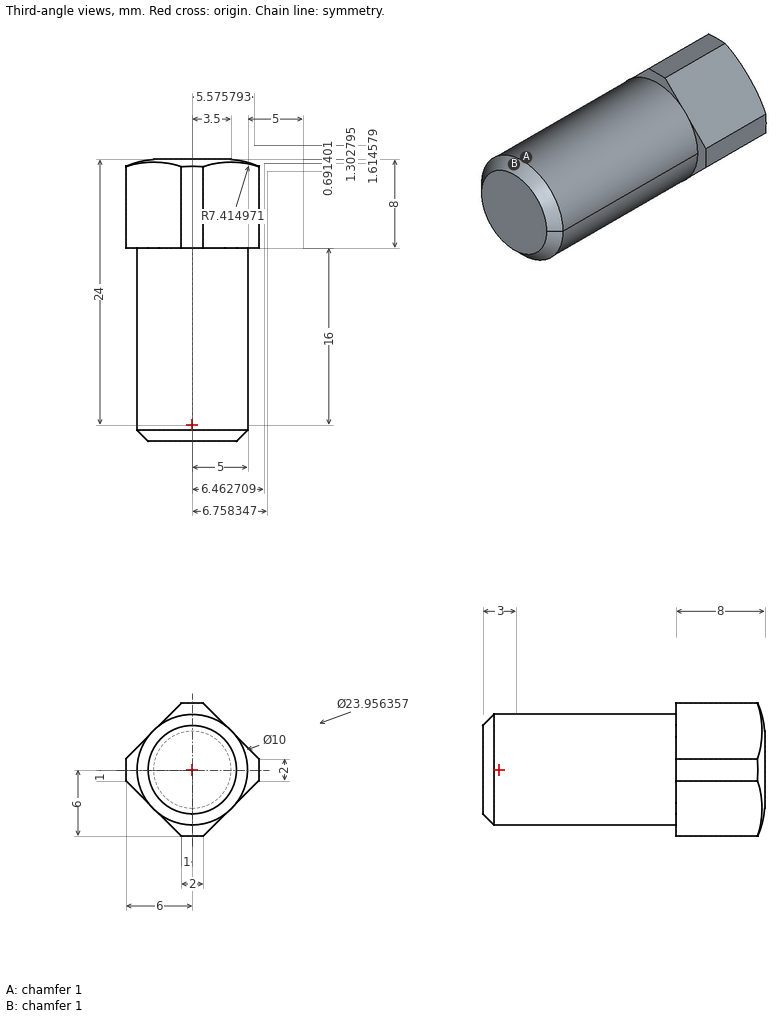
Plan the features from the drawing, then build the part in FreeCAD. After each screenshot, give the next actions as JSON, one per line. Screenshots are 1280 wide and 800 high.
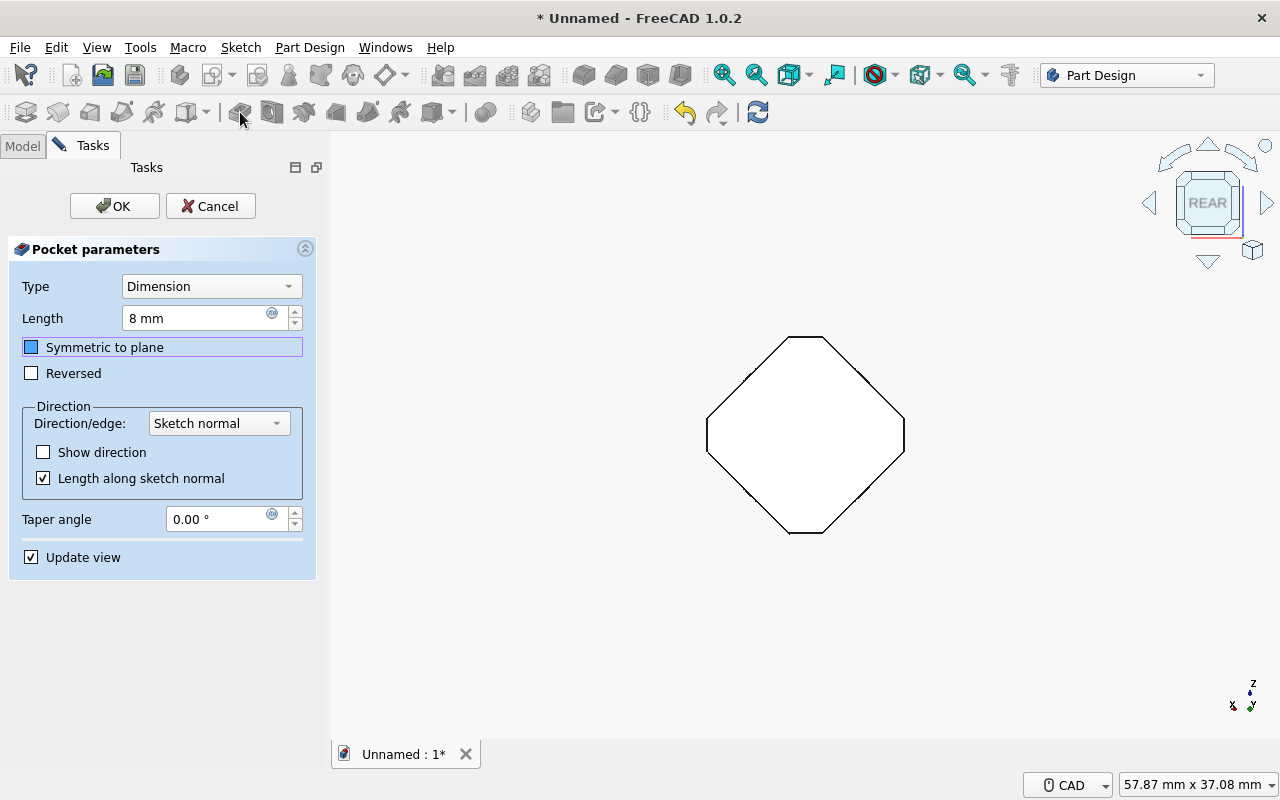
{"action": "left_click", "coordinate": [115, 206]}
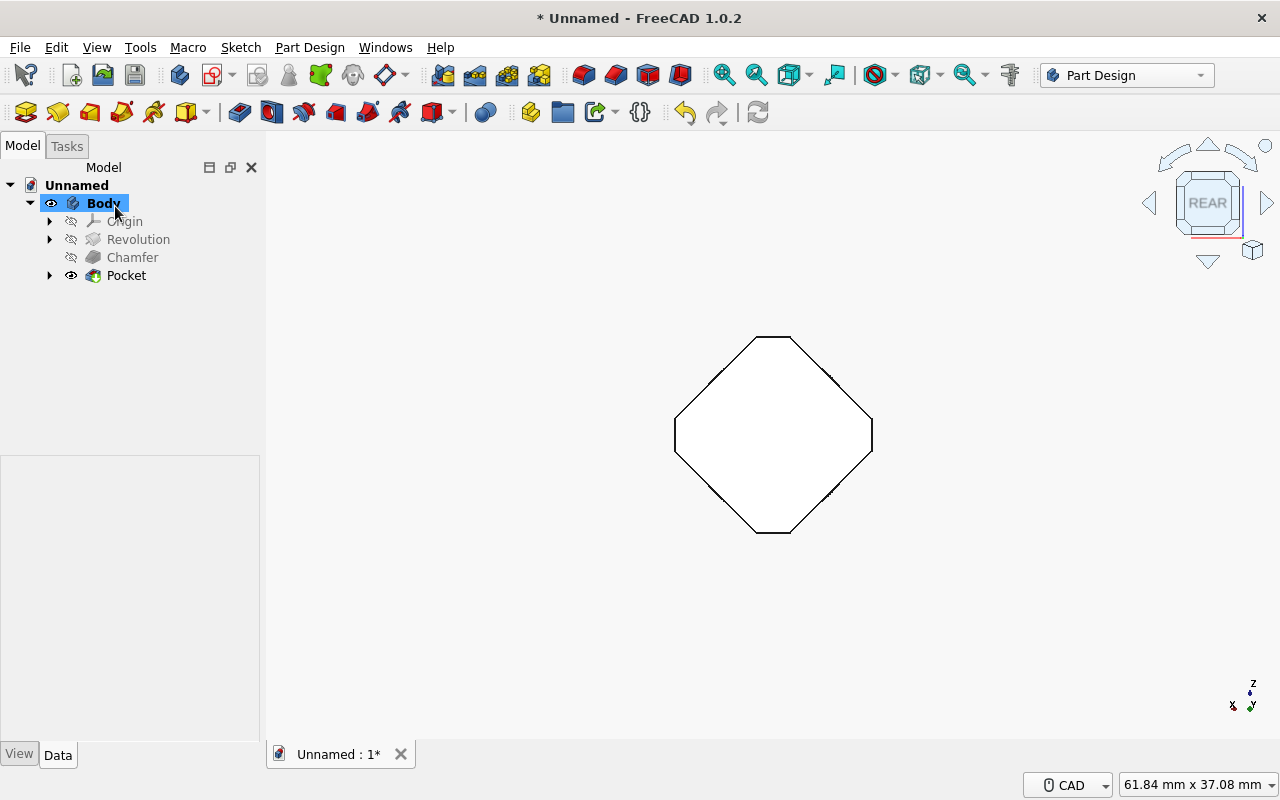
{"action": "left_click", "coordinate": [726, 76]}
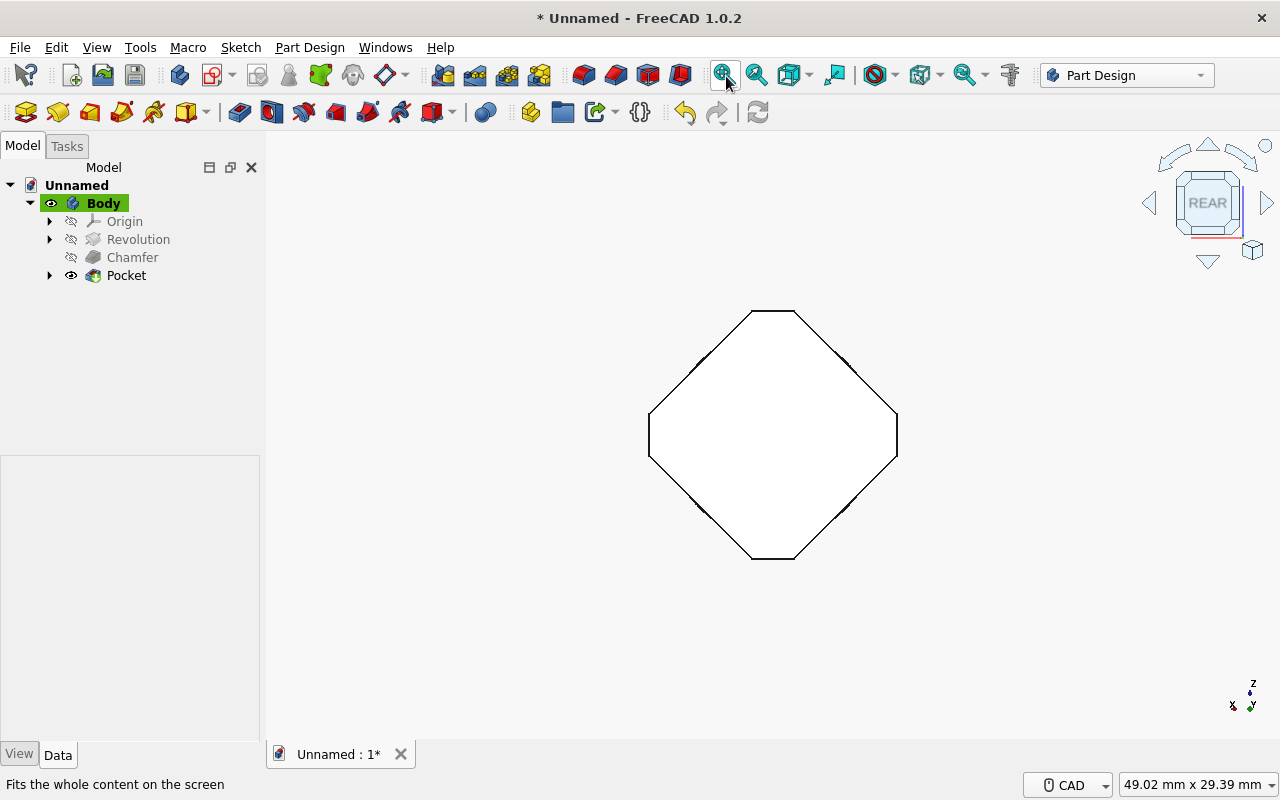
{"action": "left_click", "coordinate": [212, 76]}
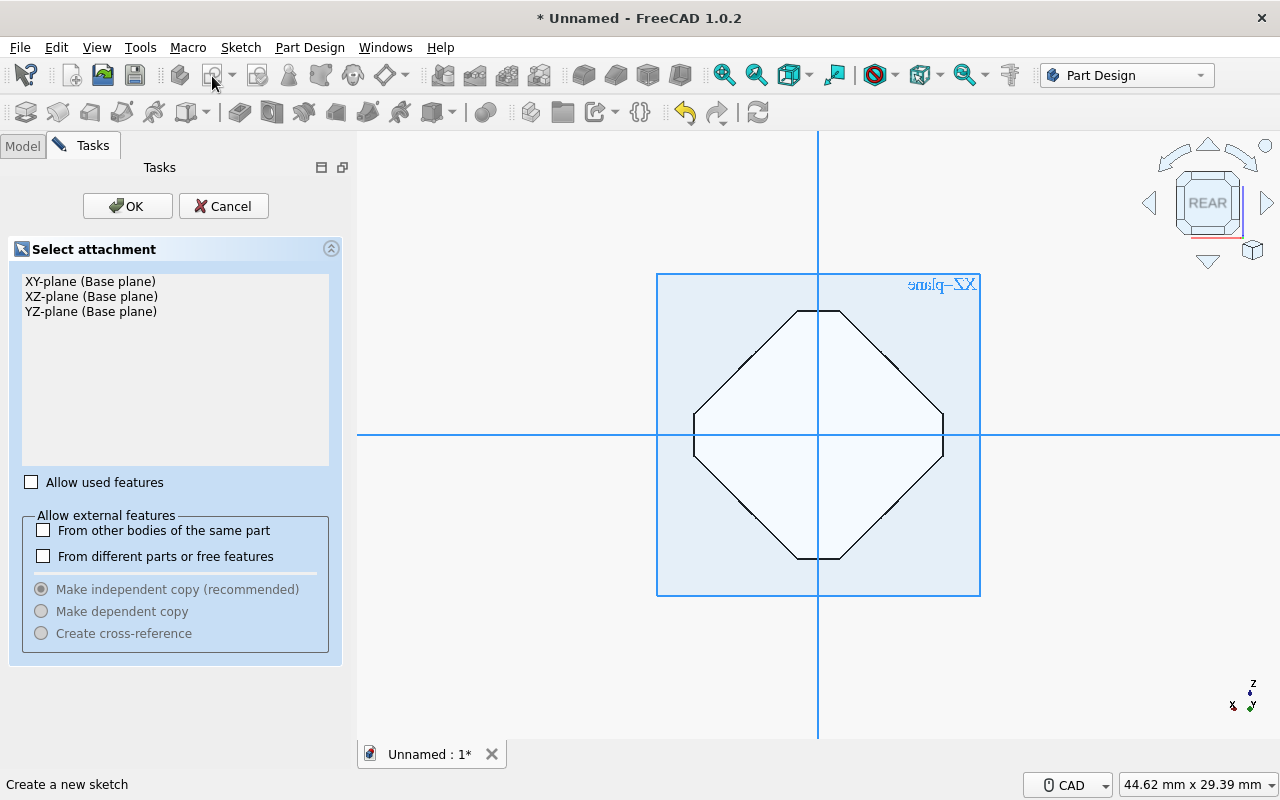
{"action": "left_click", "coordinate": [82, 282]}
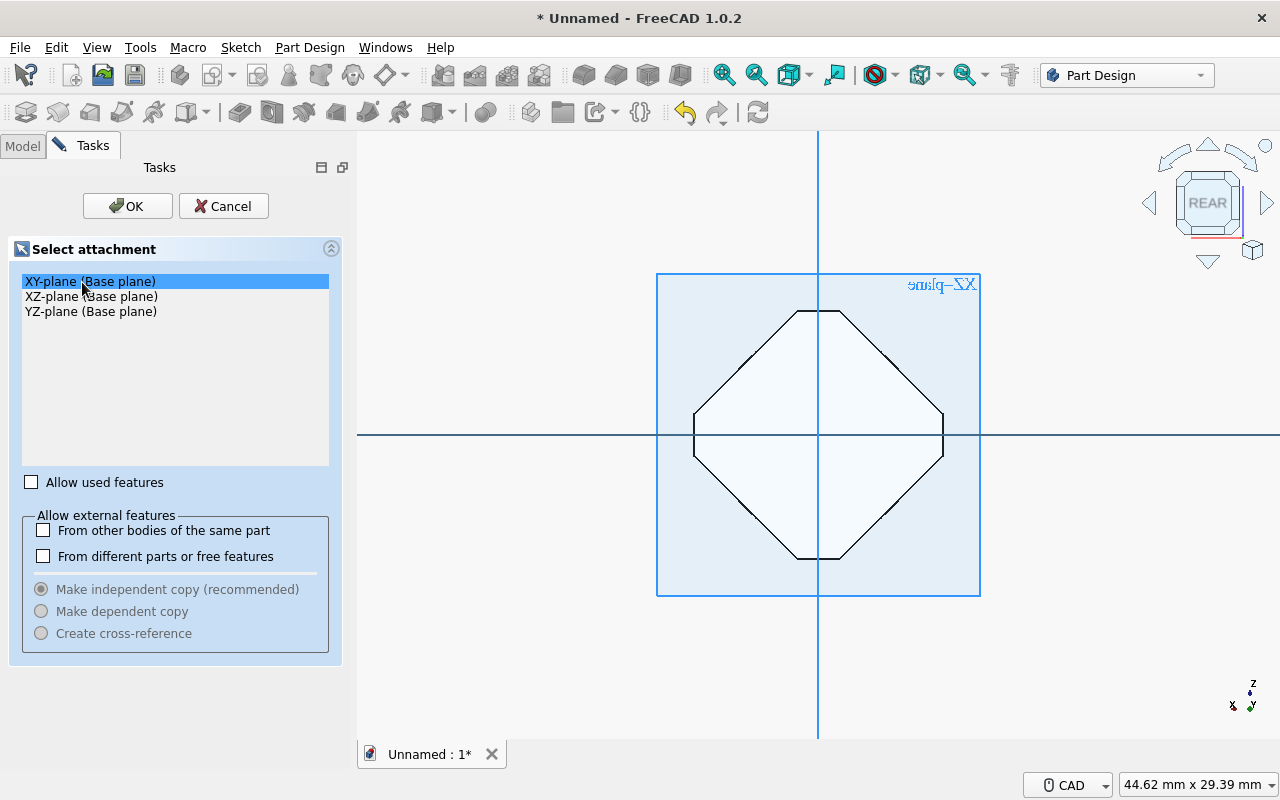
{"action": "left_click", "coordinate": [128, 206]}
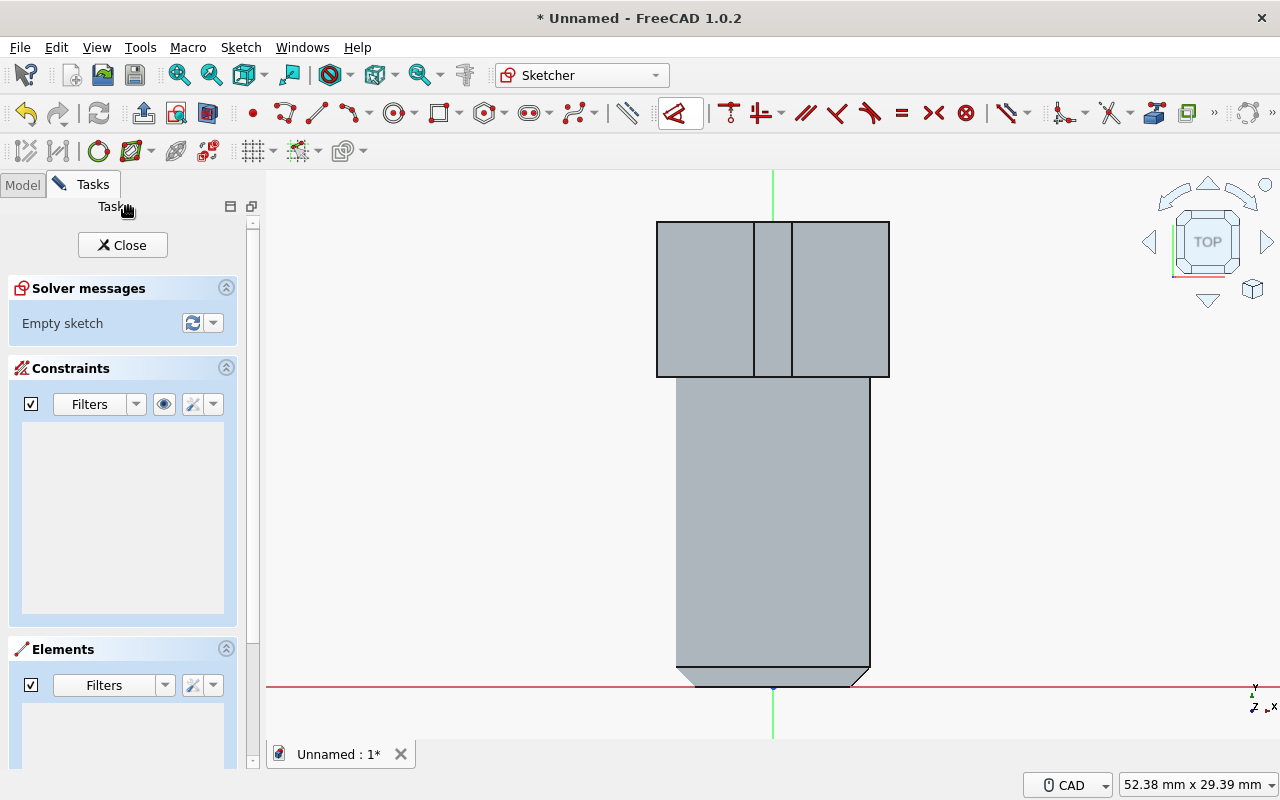
{"action": "left_click", "coordinate": [208, 114]}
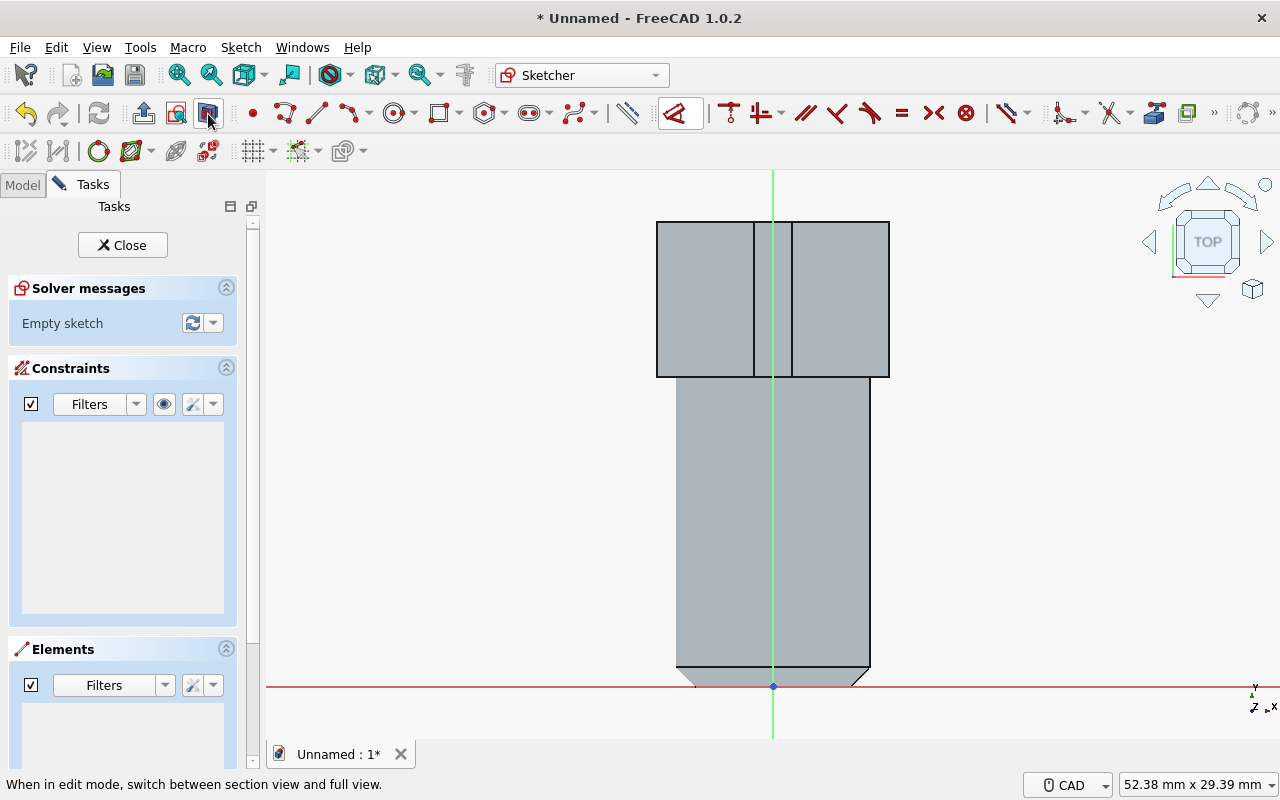
{"action": "scroll", "coordinate": [704, 454], "scroll_direction": "down", "scroll_amount": 5}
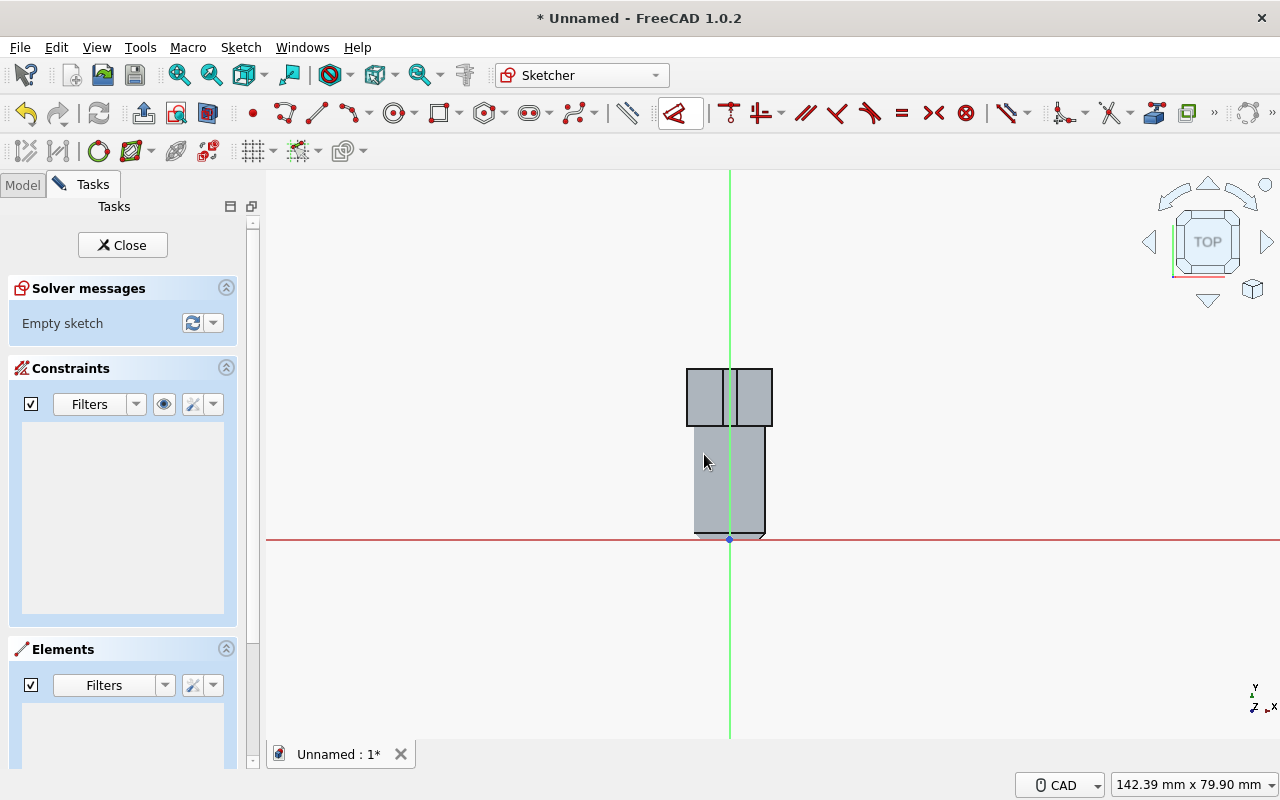
{"action": "scroll", "coordinate": [769, 363], "scroll_direction": "up", "scroll_amount": 15}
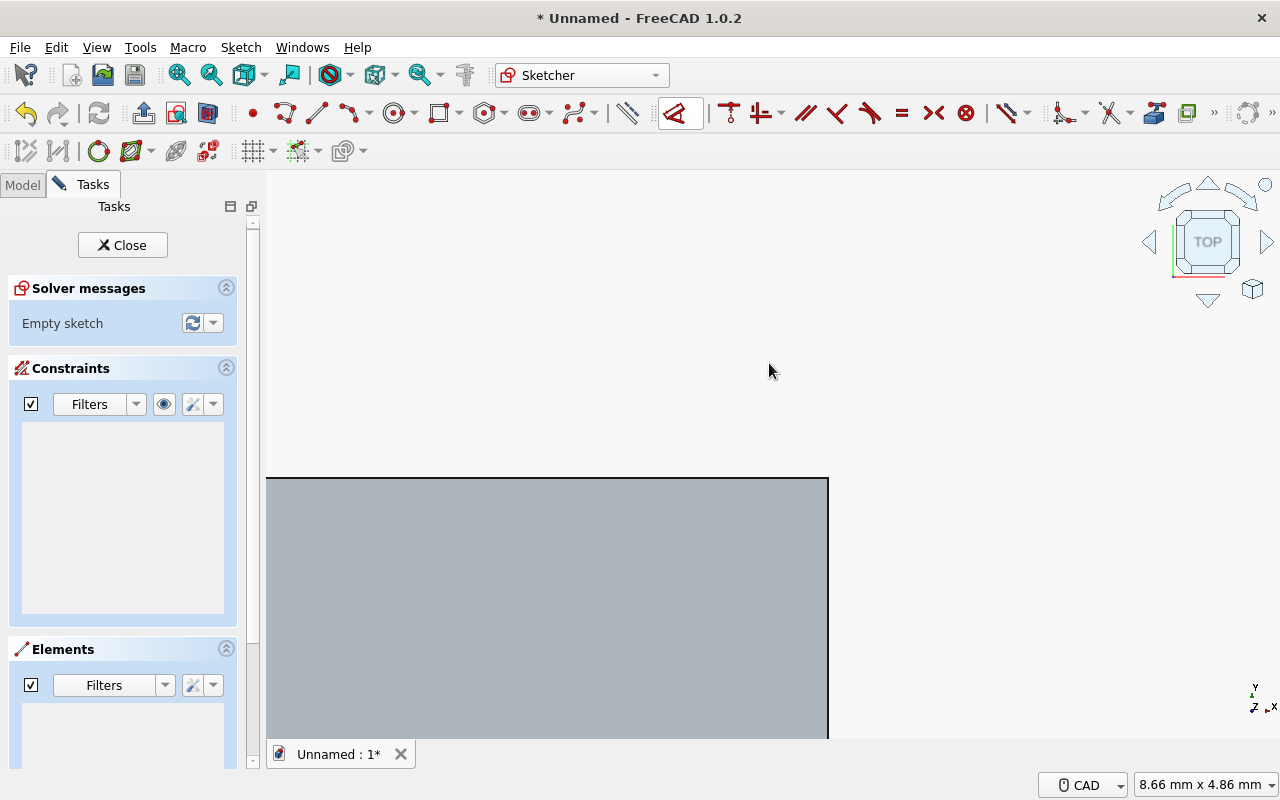
{"action": "left_click", "coordinate": [286, 114]}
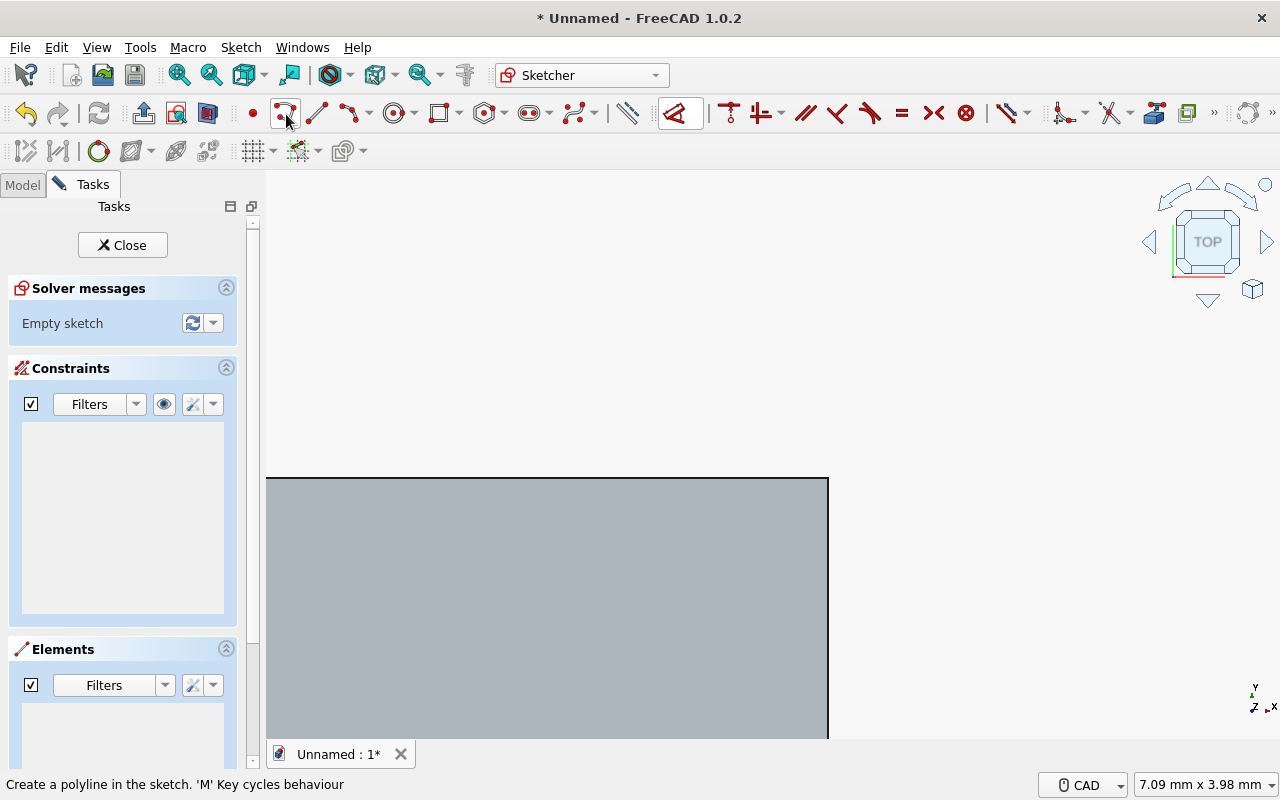
{"action": "left_click", "coordinate": [936, 621]}
{"action": "left_click", "coordinate": [894, 523]}
{"action": "left_click", "coordinate": [767, 292]}
{"action": "left_click", "coordinate": [470, 478]}
{"action": "right_click", "coordinate": [470, 478]}